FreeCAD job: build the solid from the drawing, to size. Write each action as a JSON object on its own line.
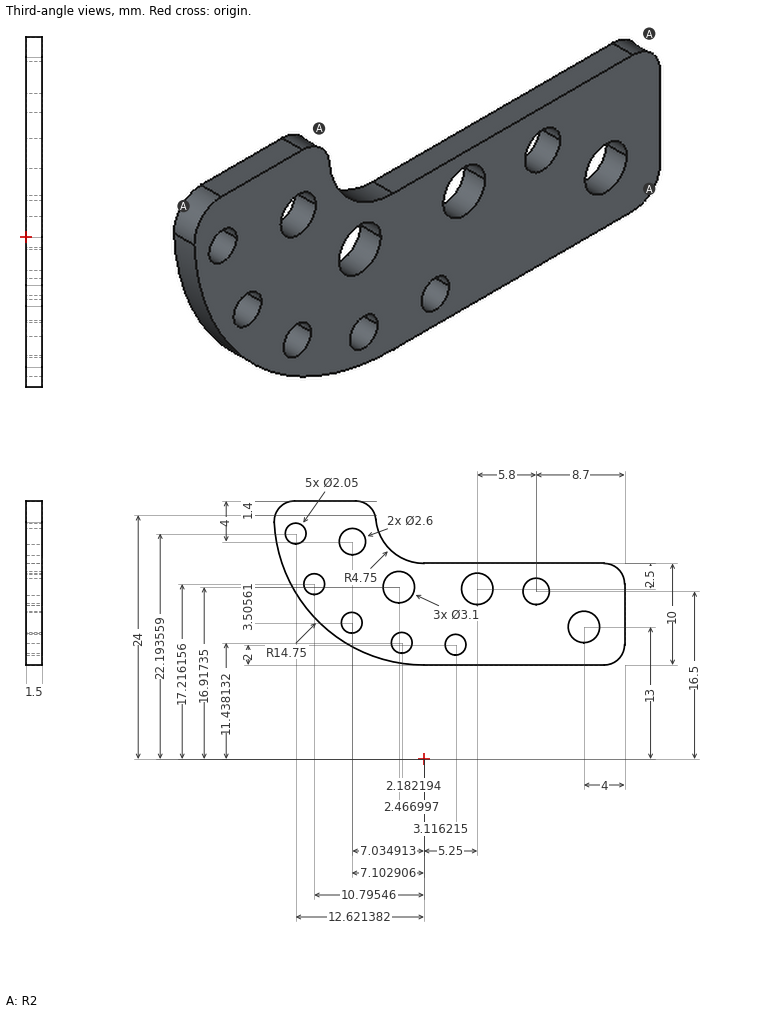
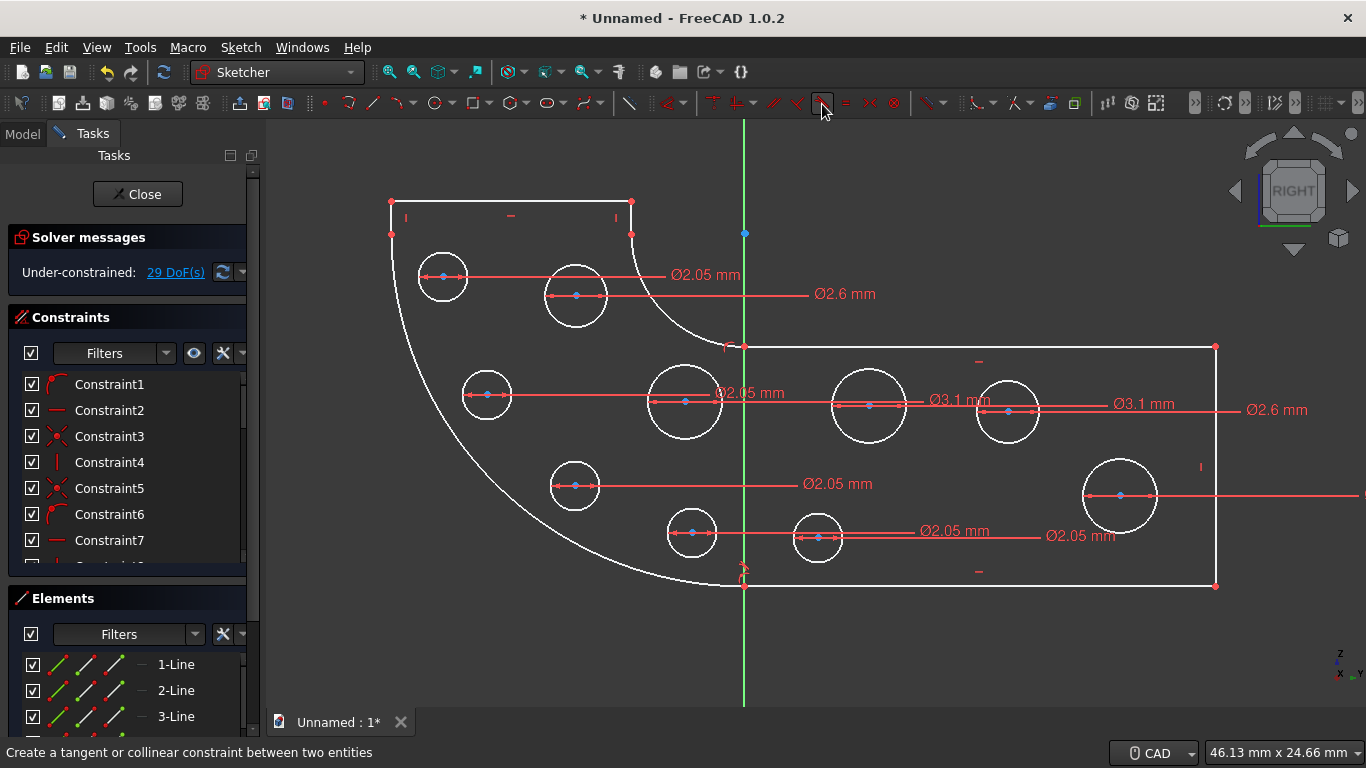
{"action": "left_click", "coordinate": [1074, 347]}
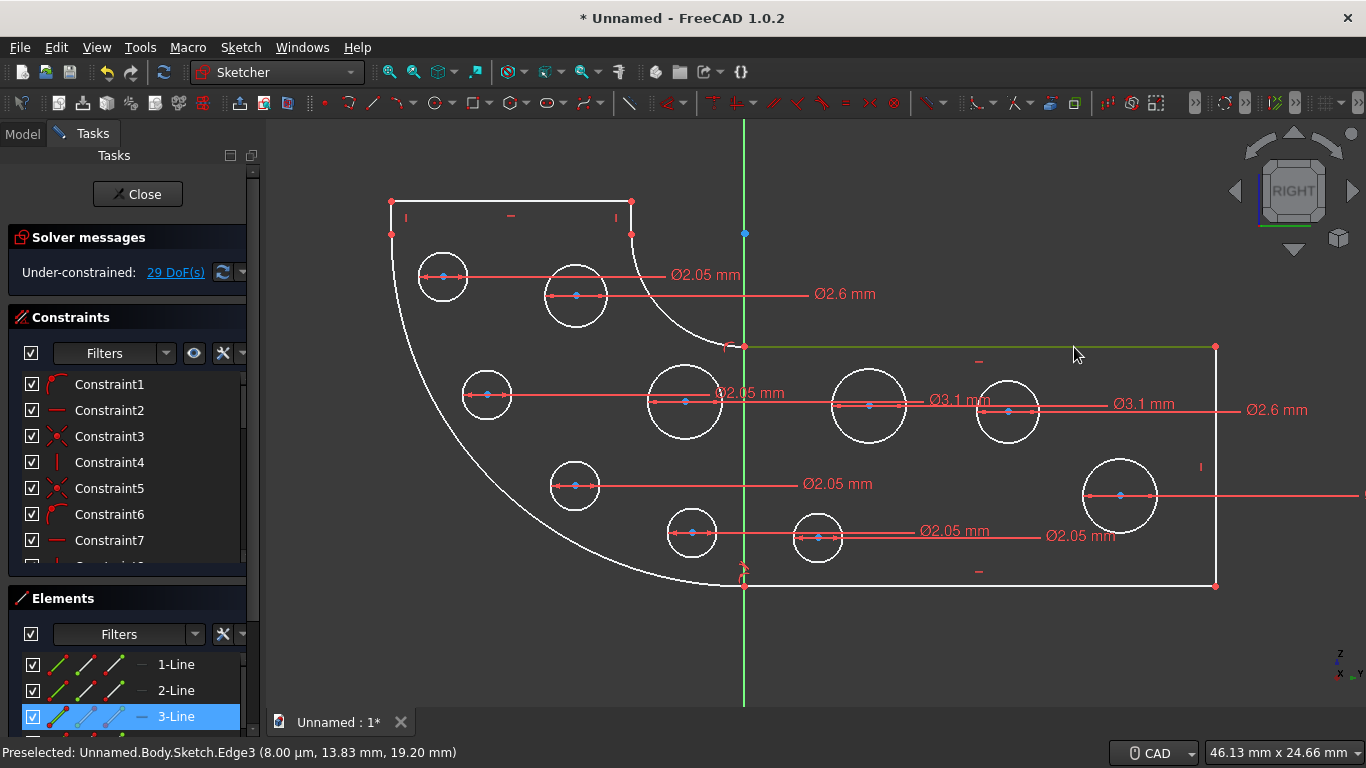
{"action": "left_click", "coordinate": [644, 285]}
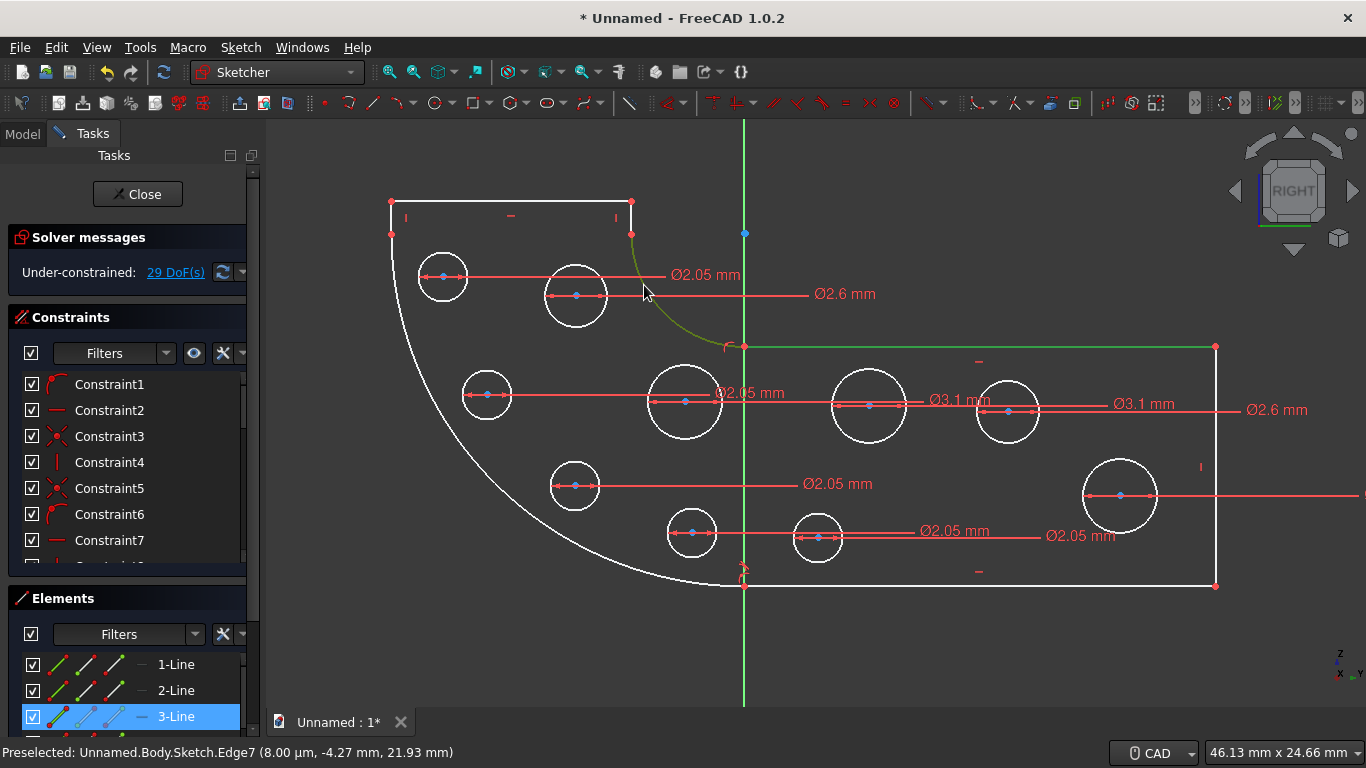
{"action": "left_click", "coordinate": [822, 104]}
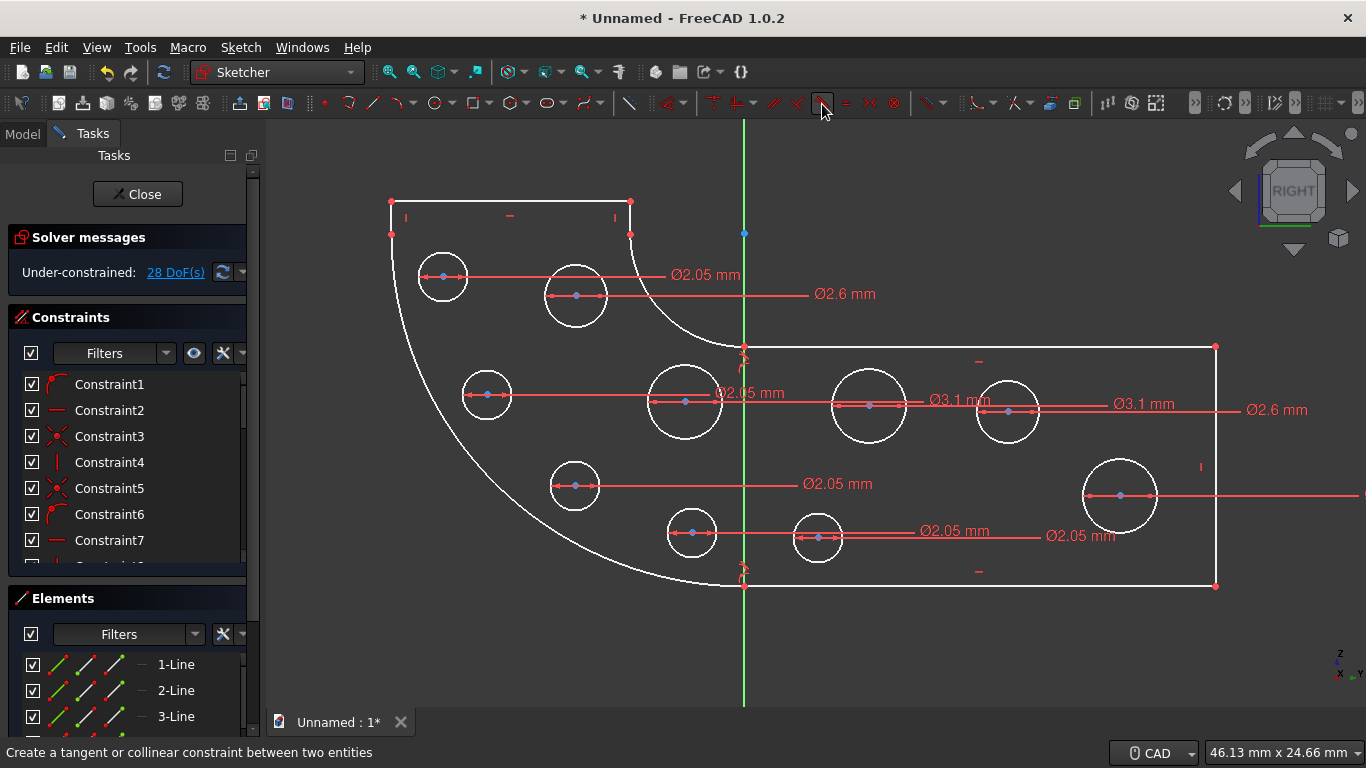
{"action": "scroll", "coordinate": [630, 224], "scroll_direction": "up", "scroll_amount": 2}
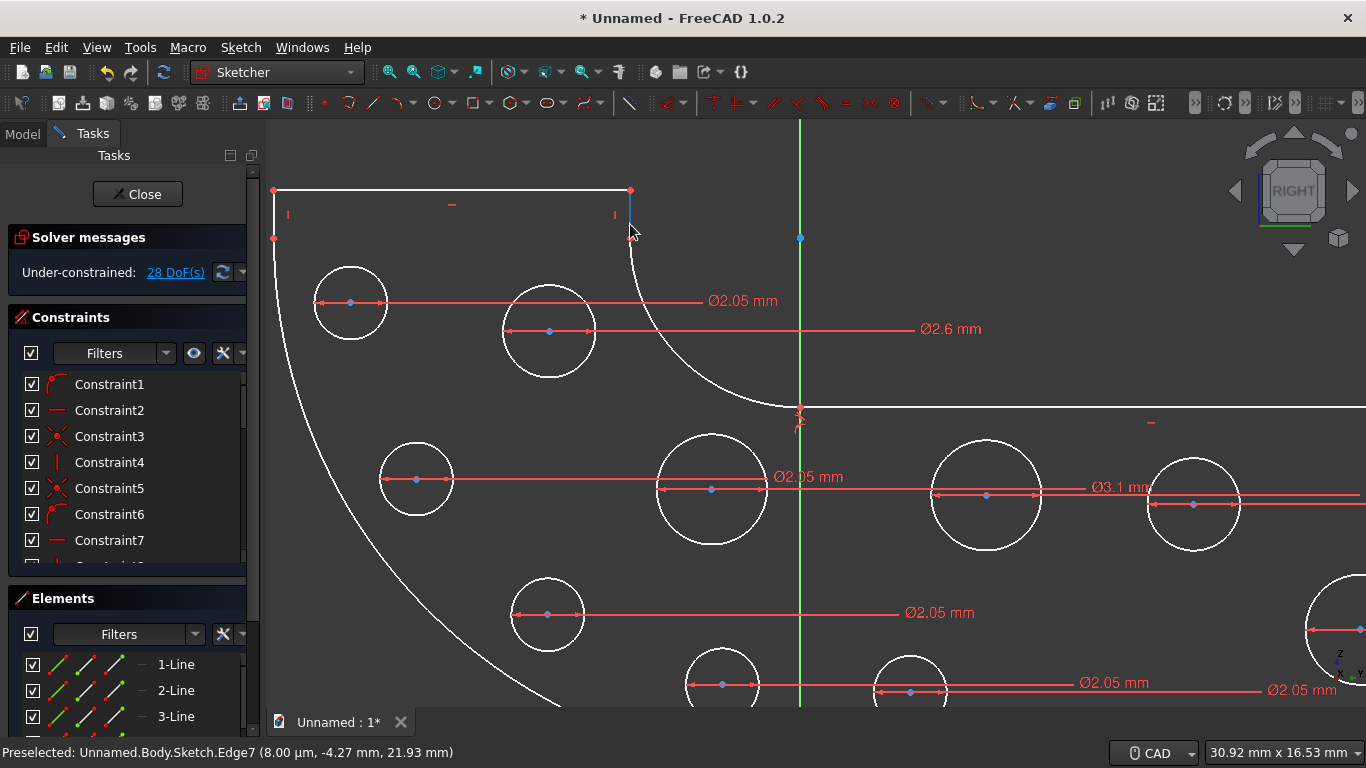
{"action": "left_click", "coordinate": [630, 224]}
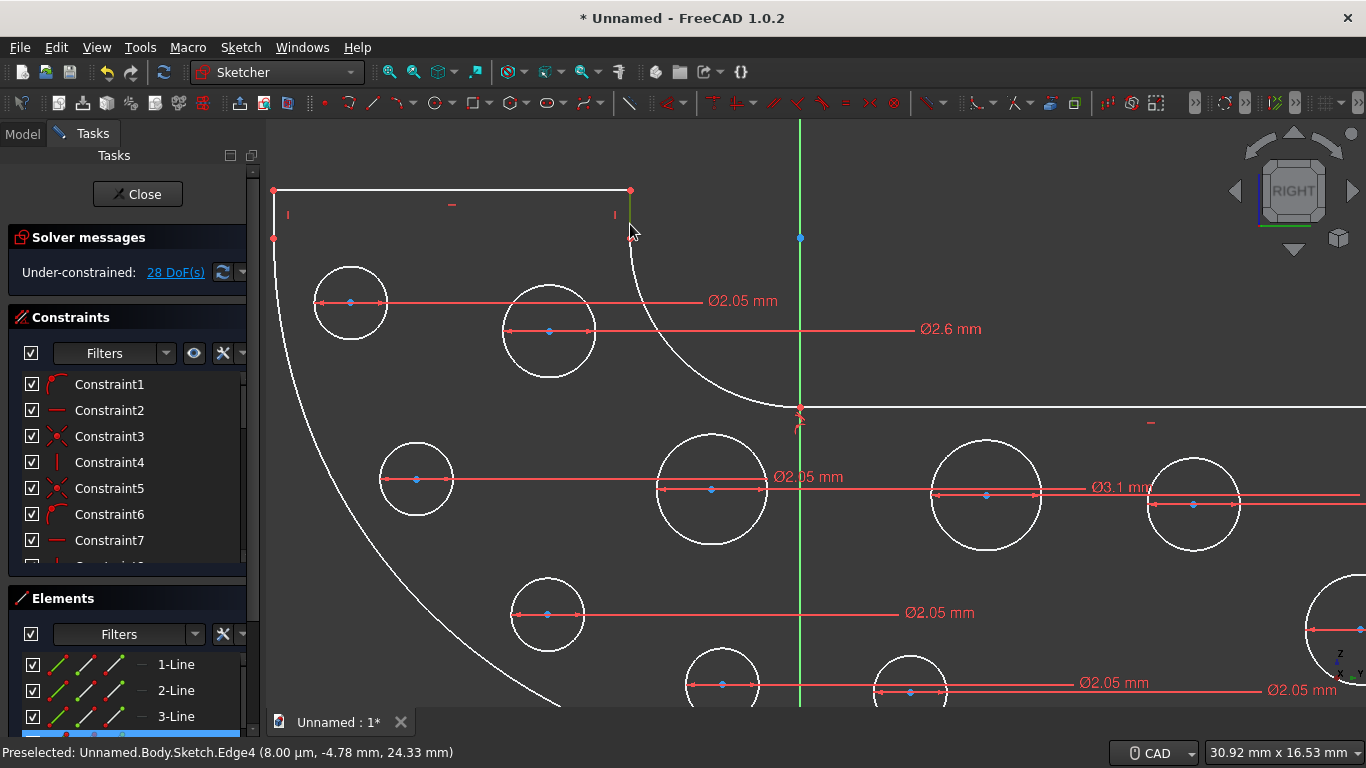
{"action": "left_click", "coordinate": [649, 315]}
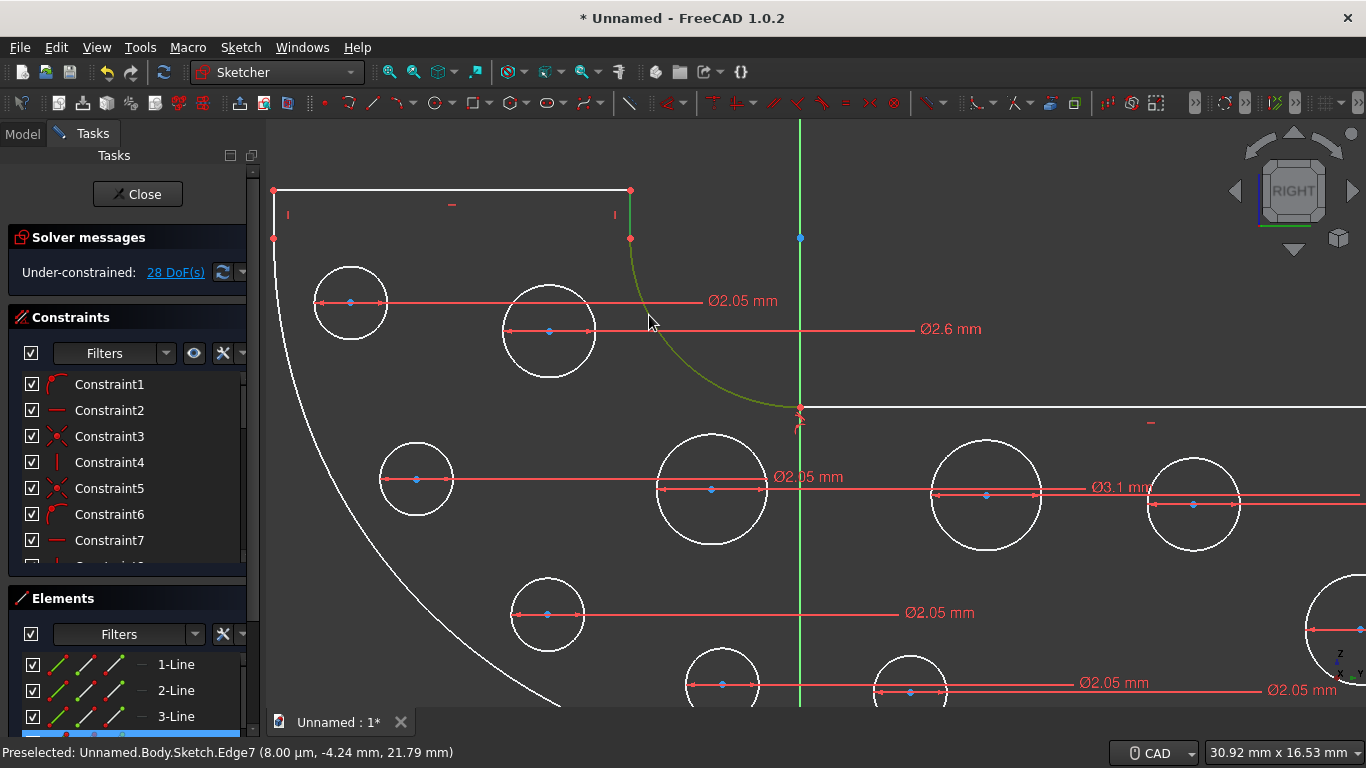
{"action": "left_click", "coordinate": [822, 104]}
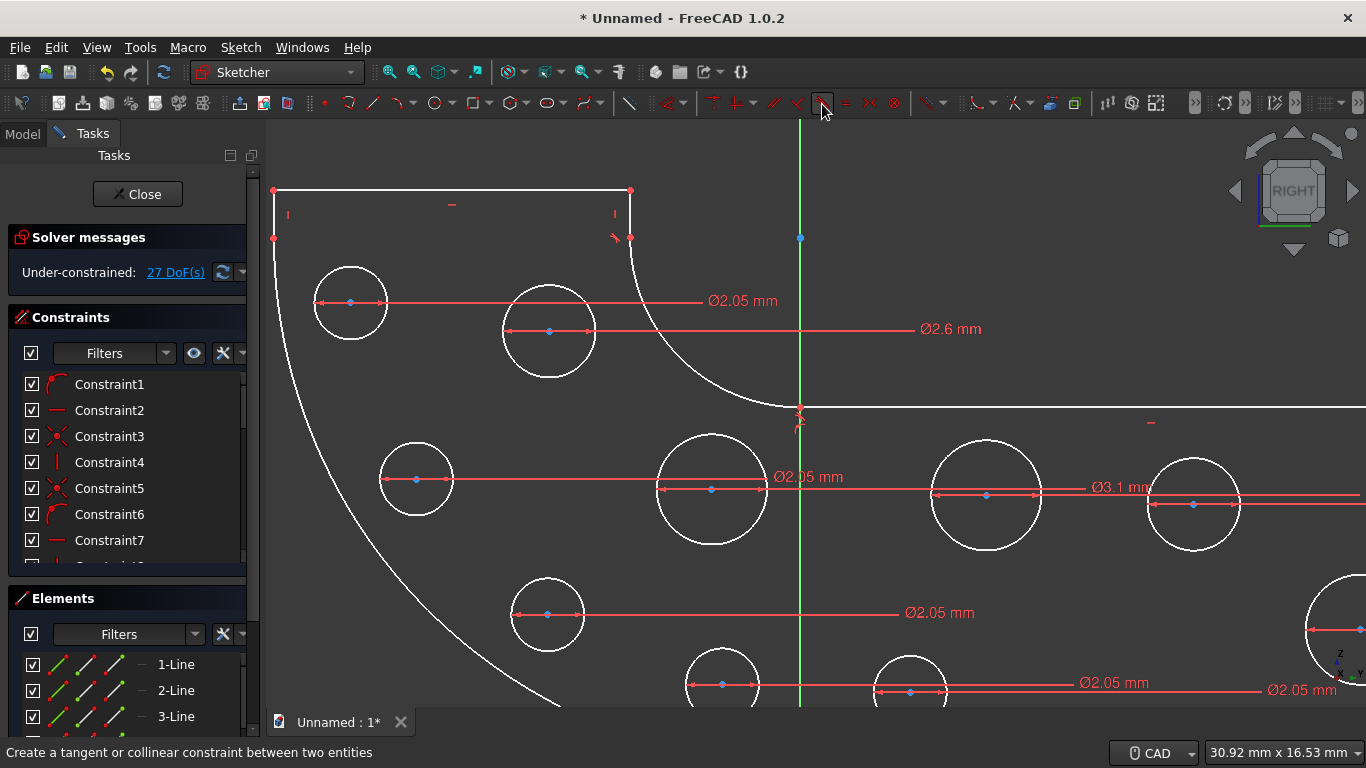
{"action": "scroll", "coordinate": [632, 229], "scroll_direction": "down", "scroll_amount": 4}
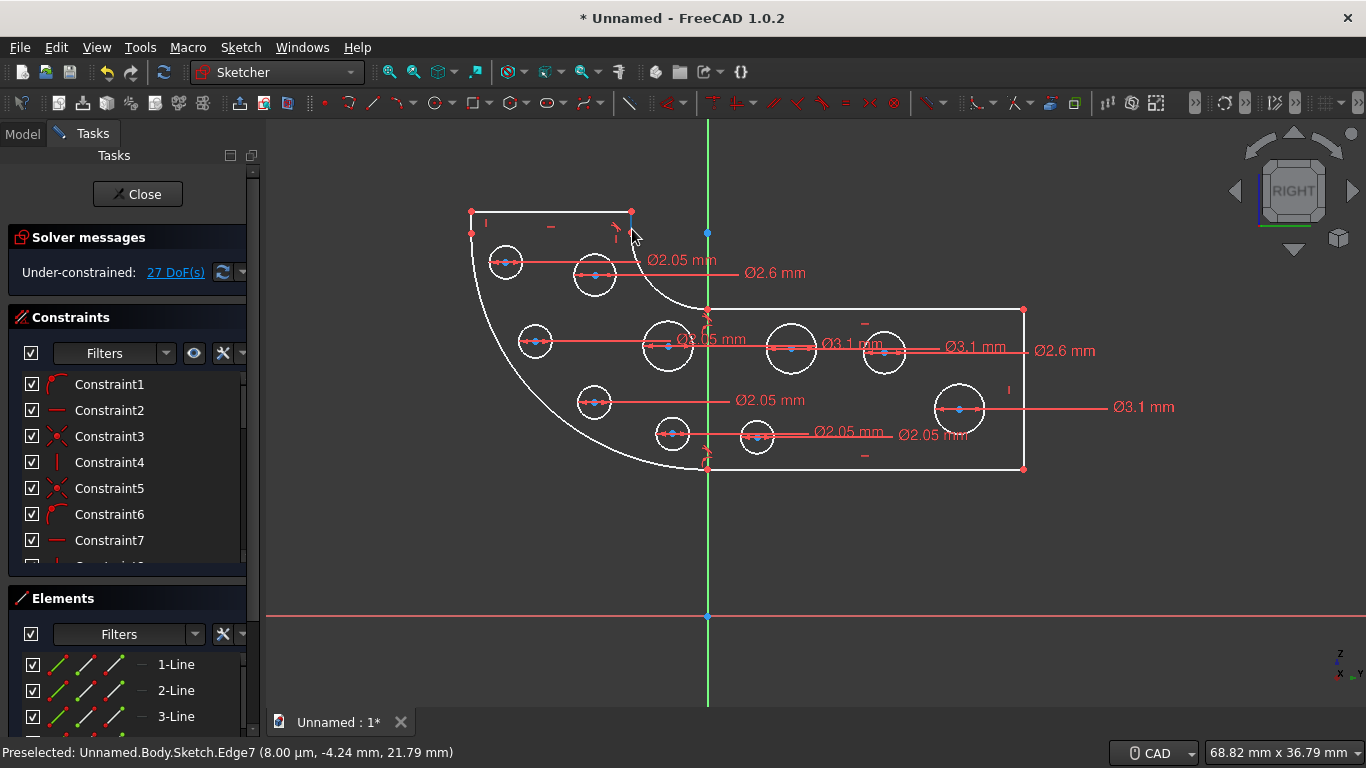
{"action": "scroll", "coordinate": [471, 218], "scroll_direction": "up", "scroll_amount": 4}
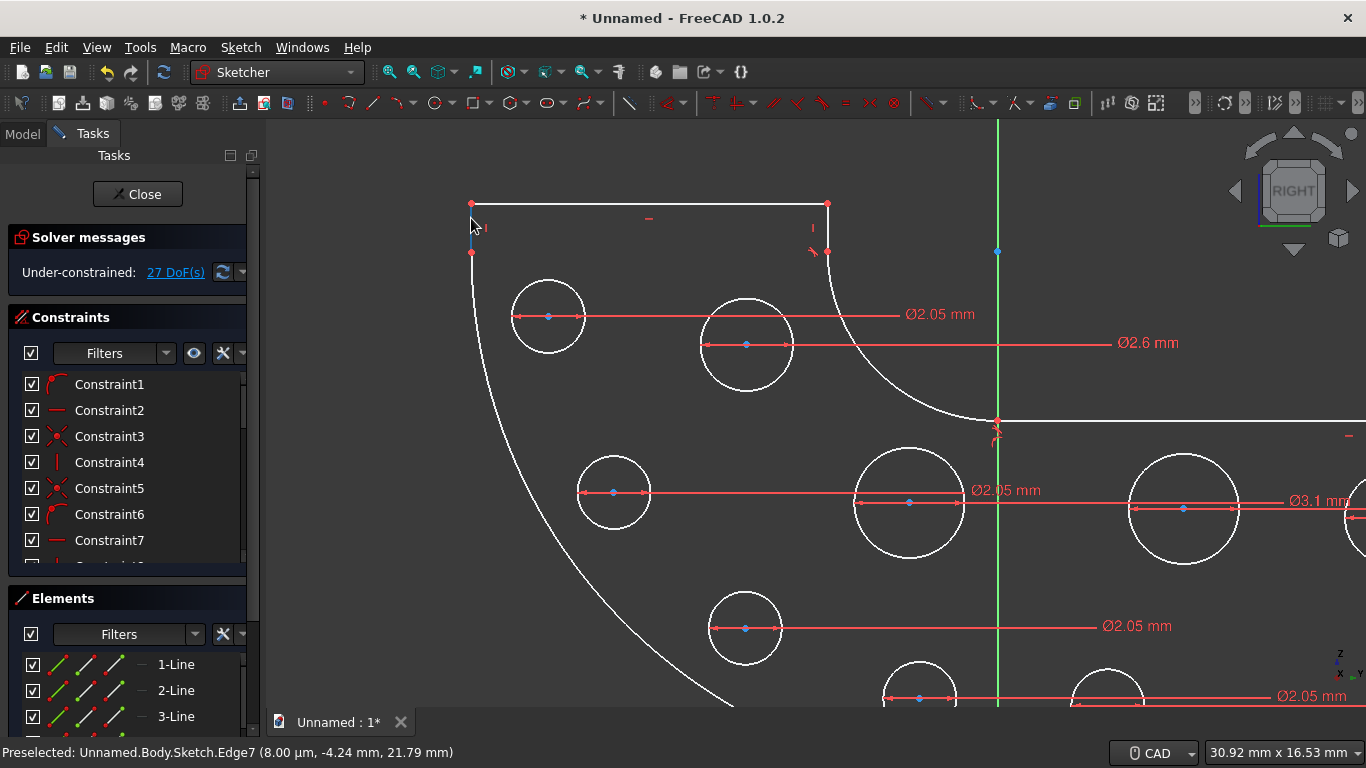
{"action": "left_click", "coordinate": [471, 218]}